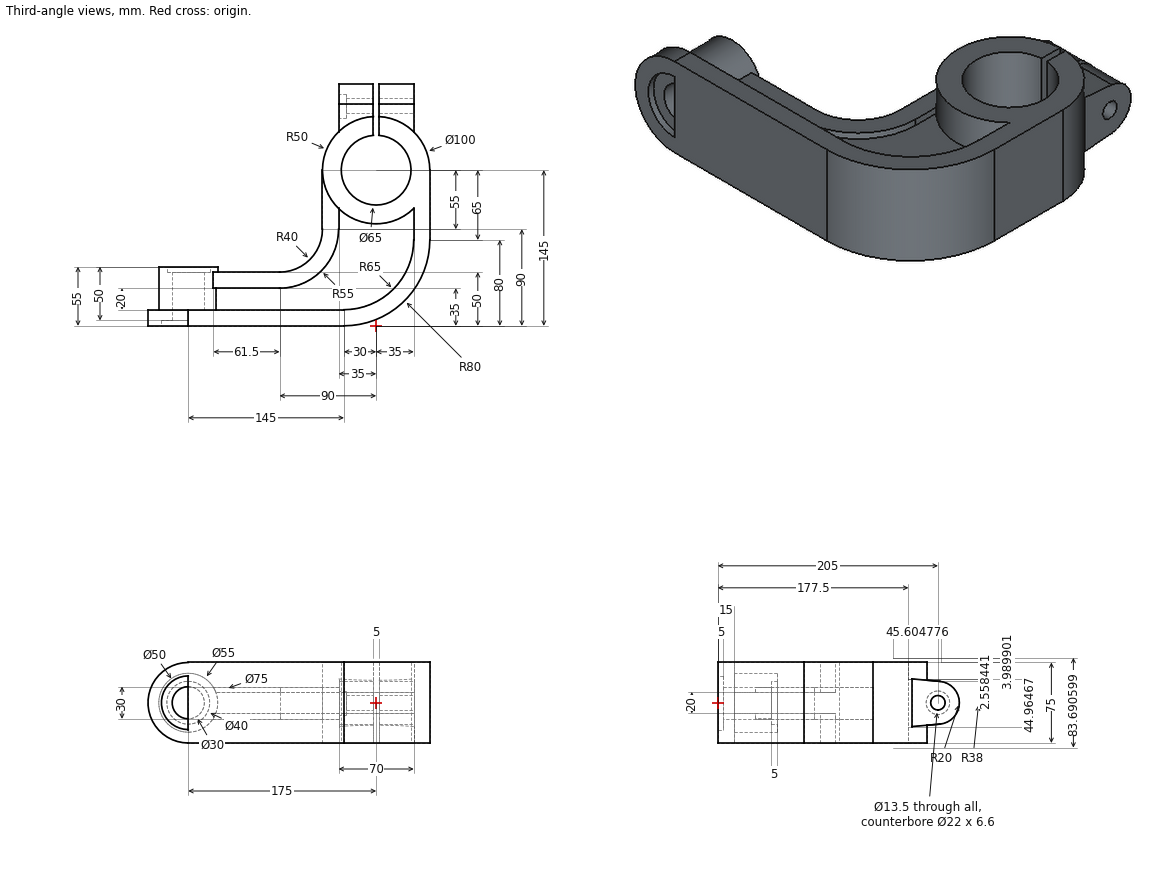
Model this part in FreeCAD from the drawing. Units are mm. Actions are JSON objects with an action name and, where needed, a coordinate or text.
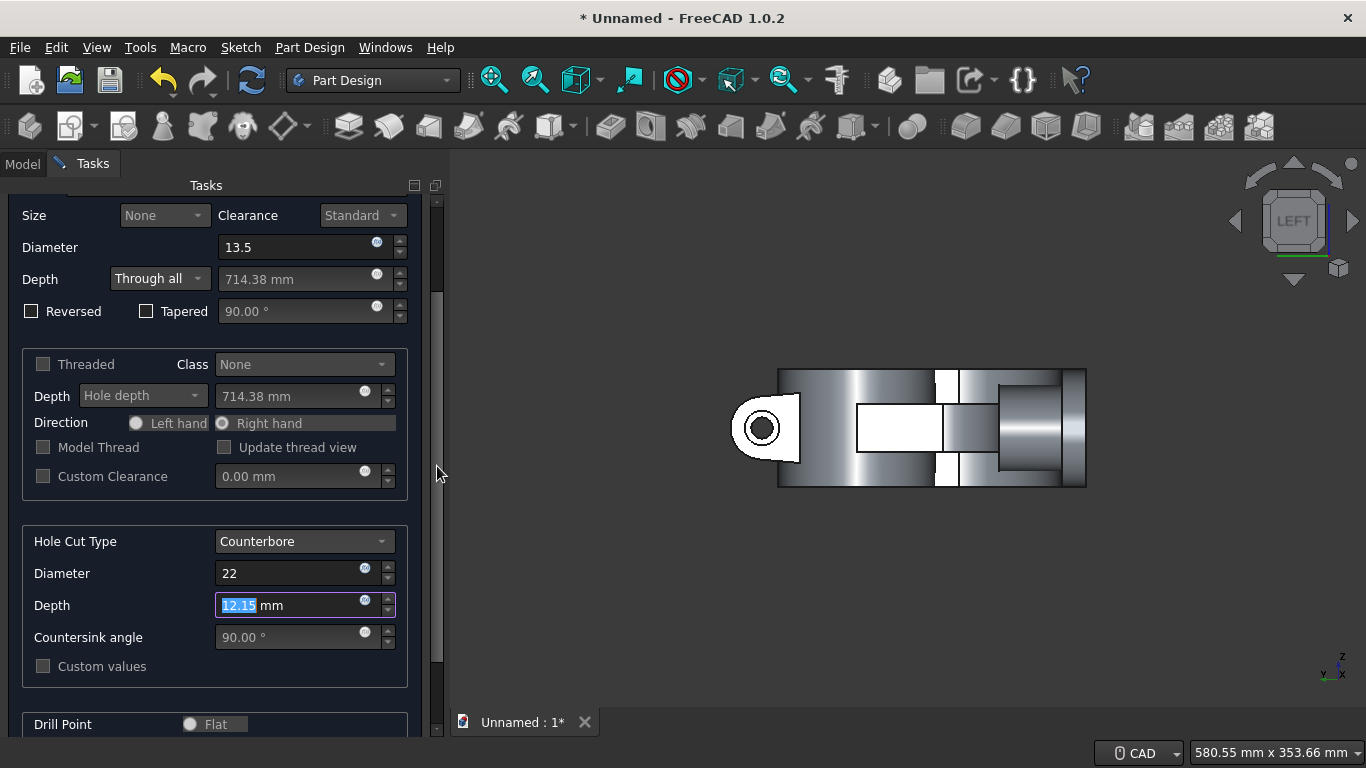
{"action": "type", "text": "6.6"}
{"action": "key", "text": "Tab"}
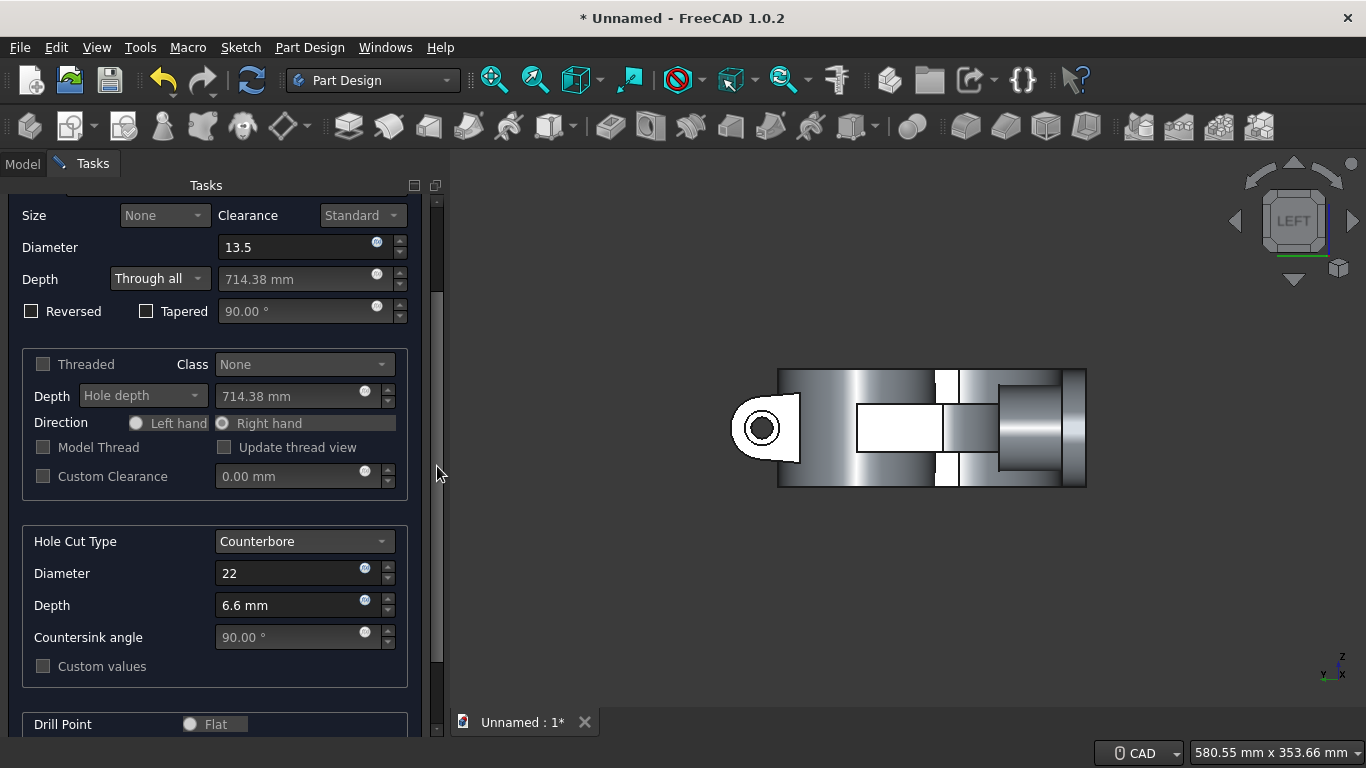
{"action": "scroll", "coordinate": [437, 466], "scroll_direction": "up", "scroll_amount": 3}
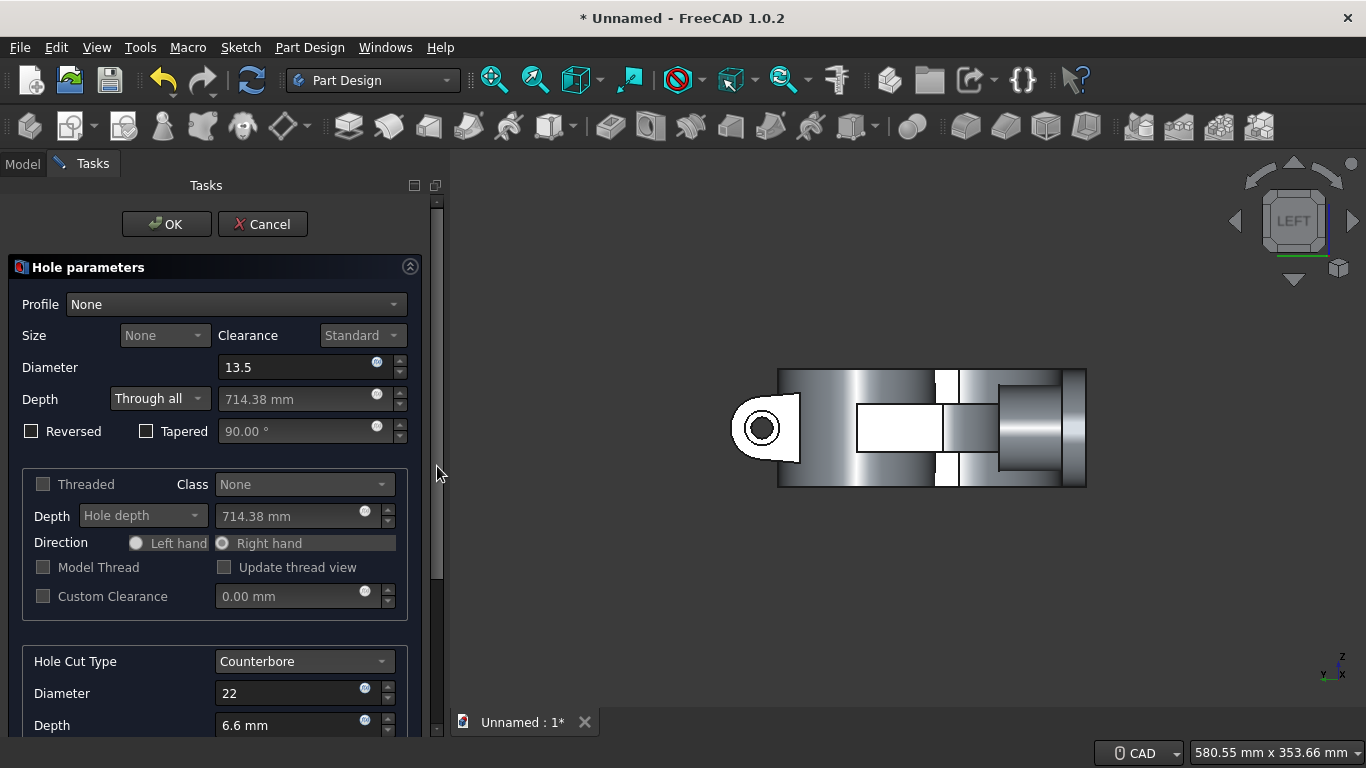
{"action": "left_click", "coordinate": [167, 224]}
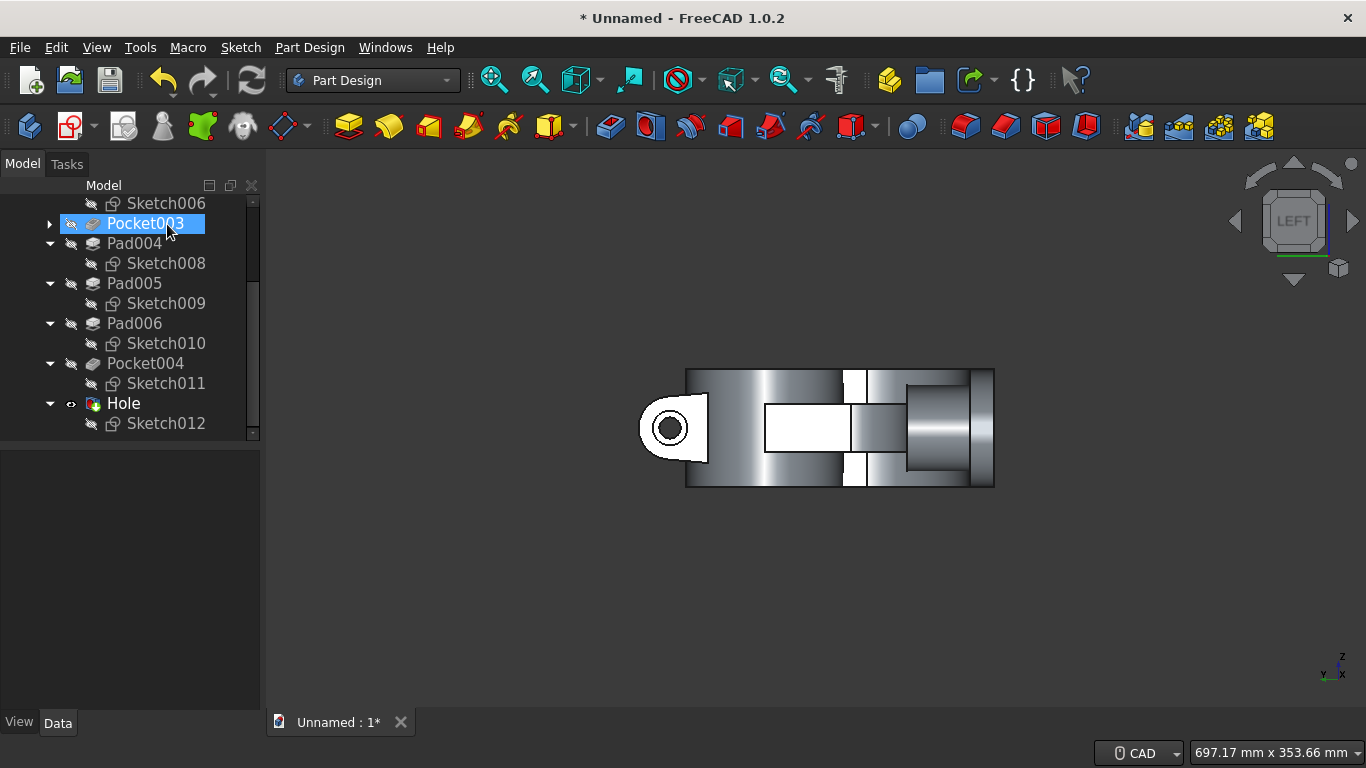
{"action": "key", "text": "0"}